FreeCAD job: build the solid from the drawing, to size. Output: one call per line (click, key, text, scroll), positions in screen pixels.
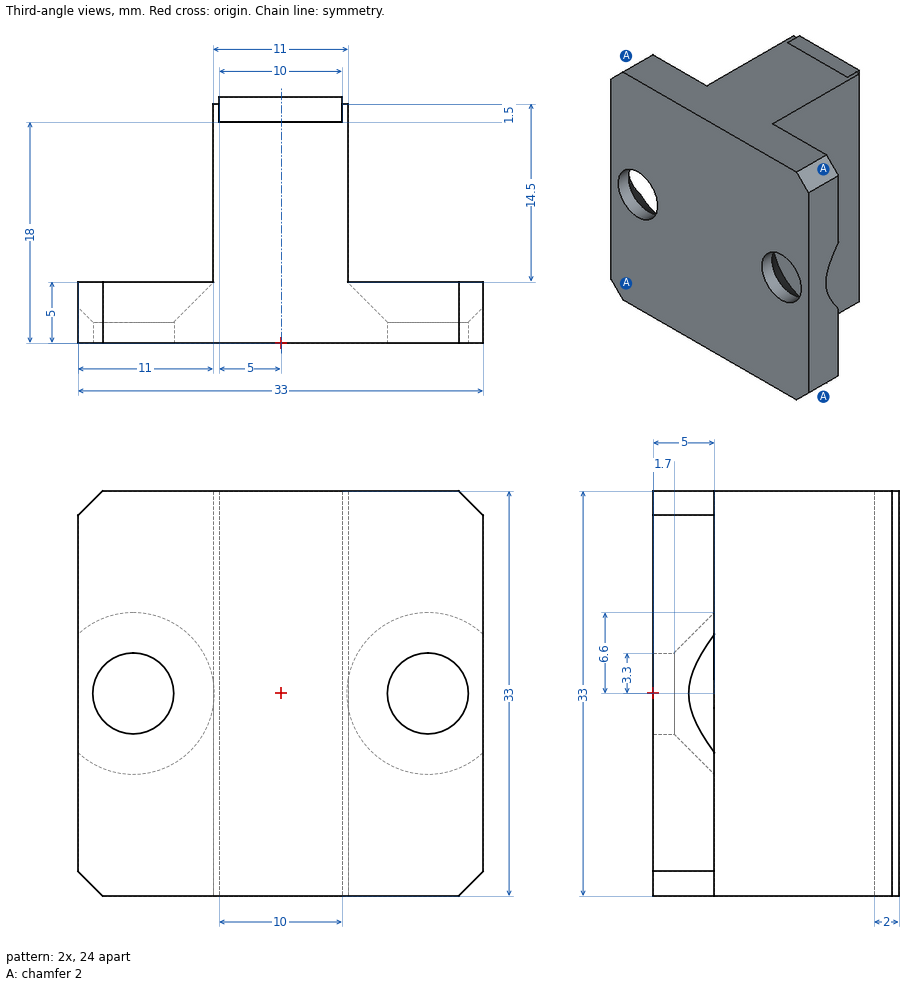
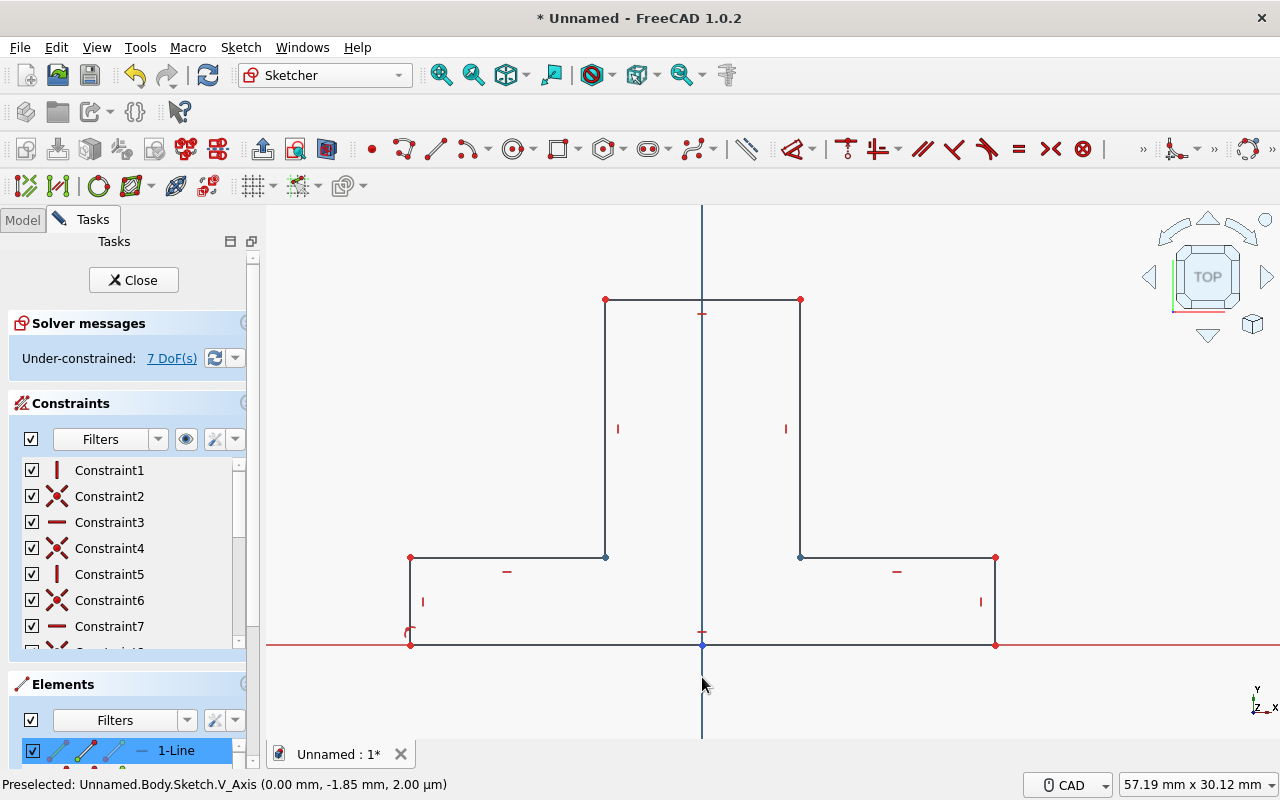
click(1052, 150)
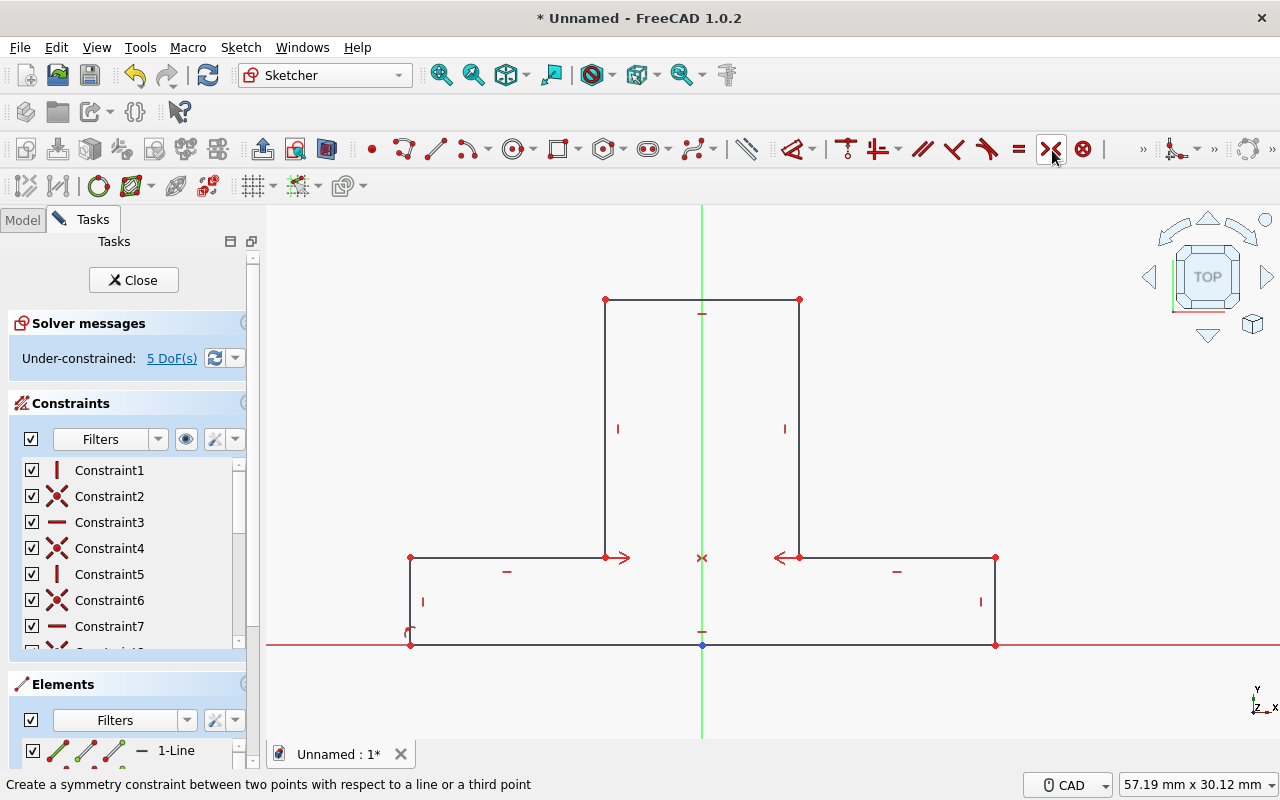
click(792, 150)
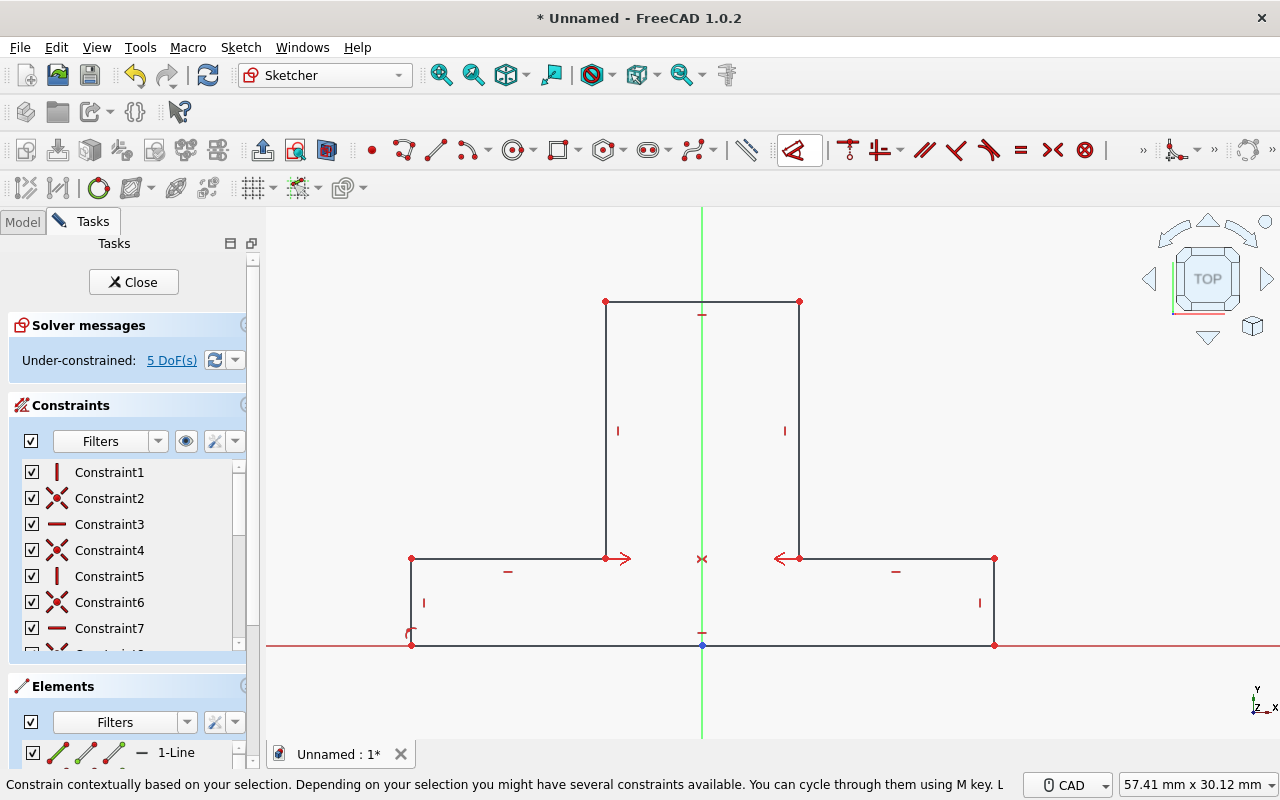
click(411, 585)
click(377, 602)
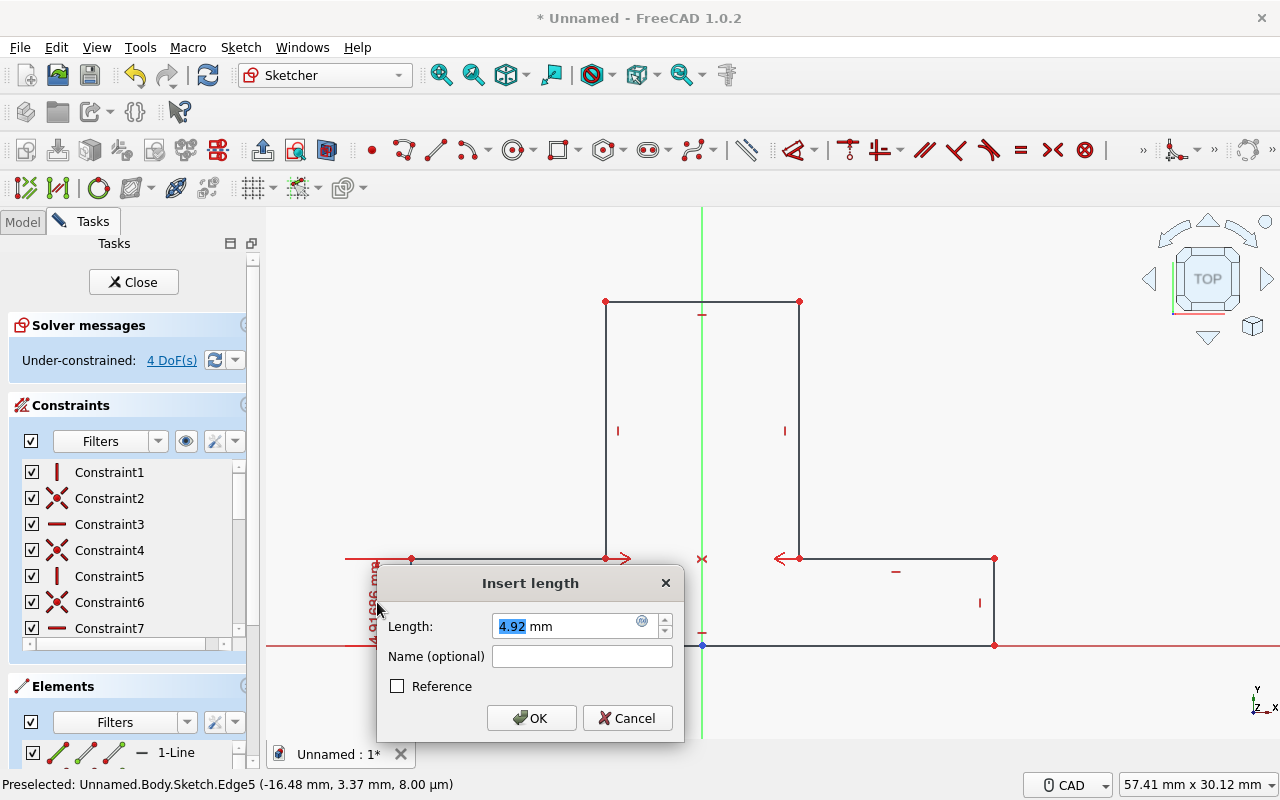
text(5)
key(Return)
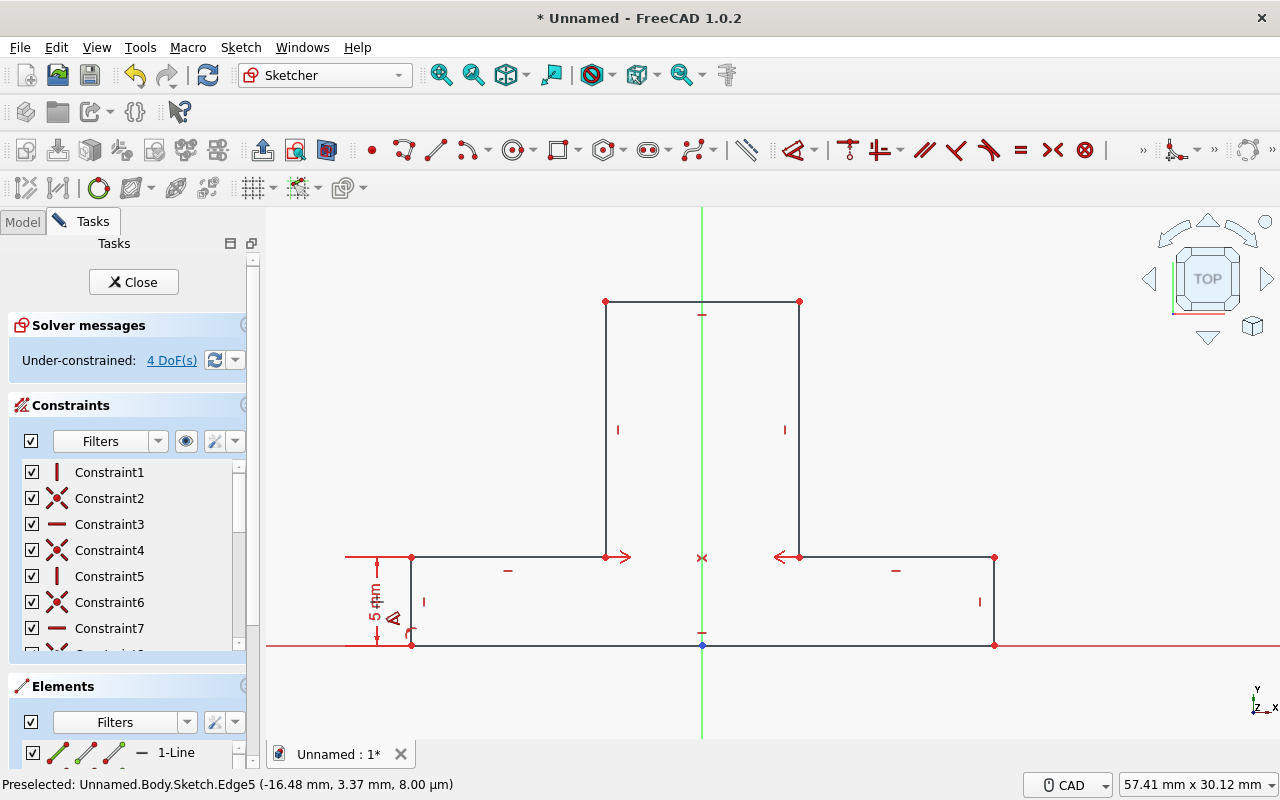
click(741, 302)
click(658, 268)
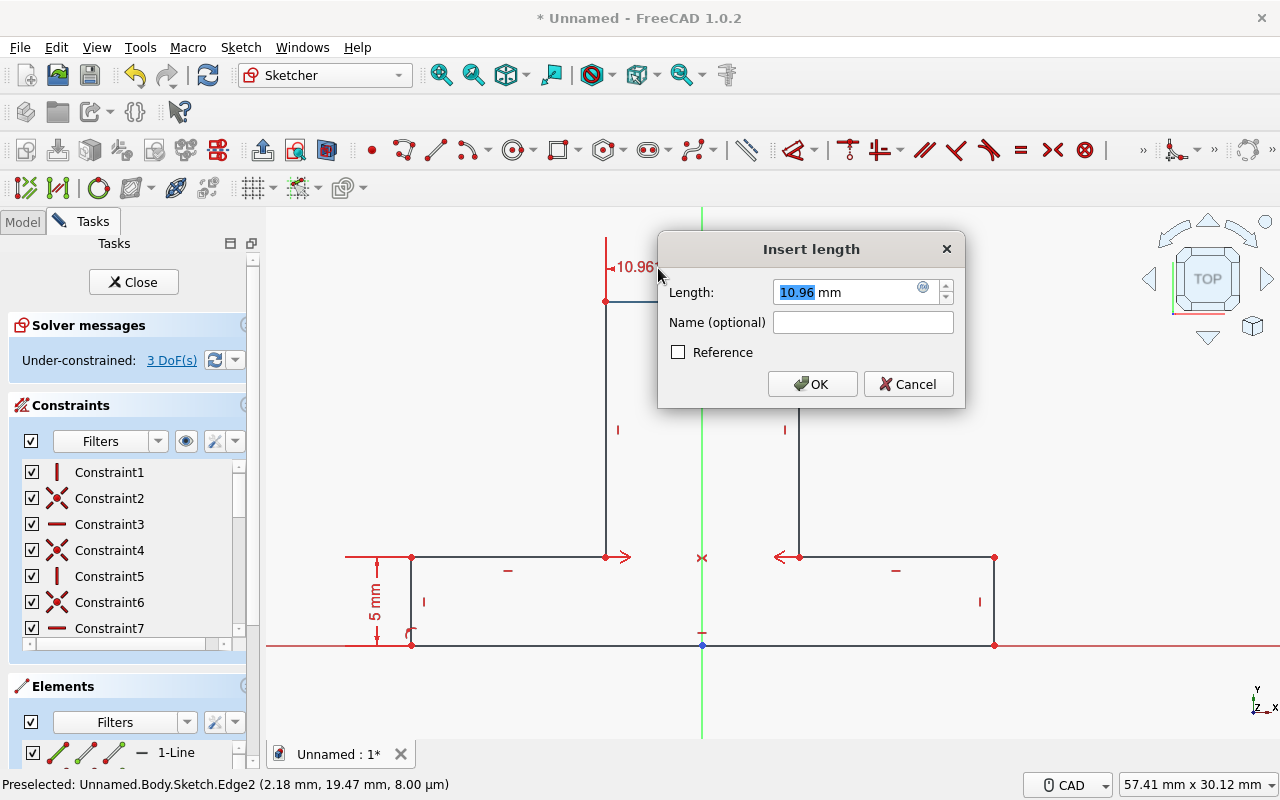
text(11)
key(Return)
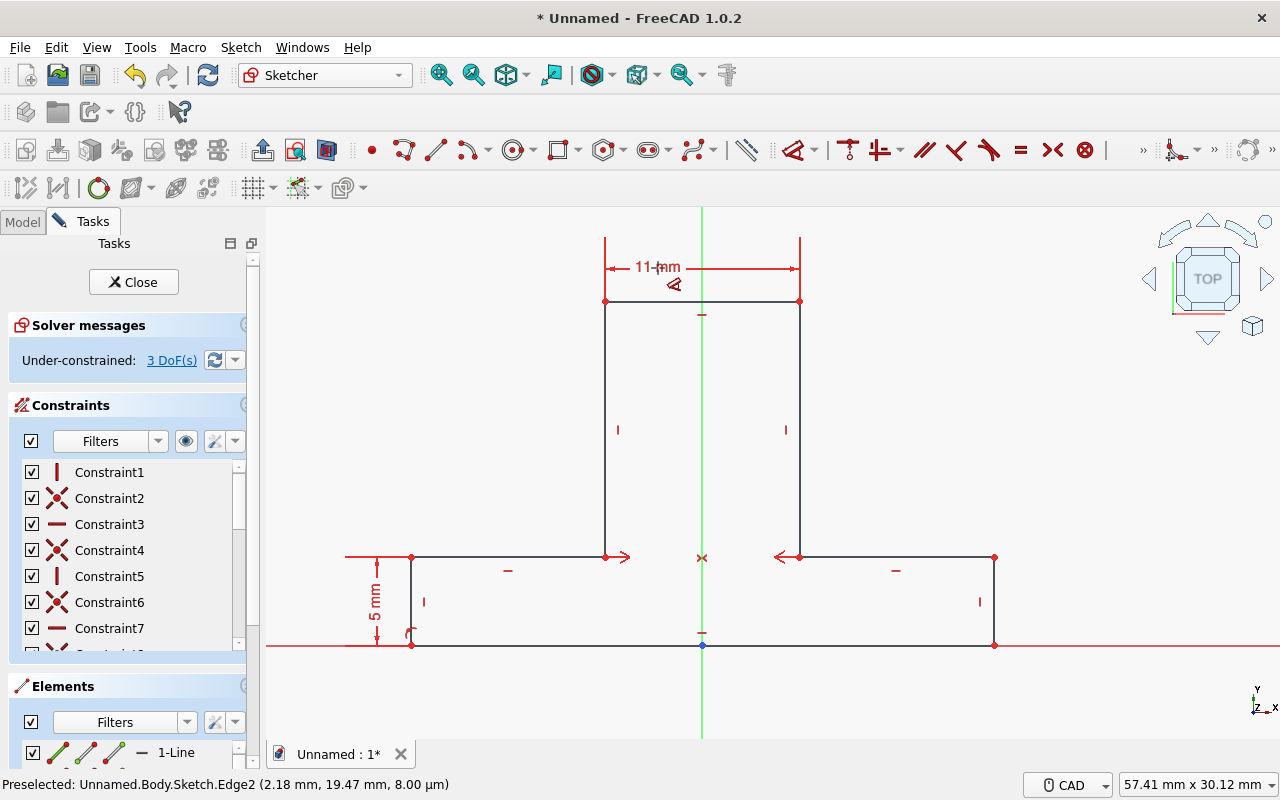
click(547, 557)
click(508, 591)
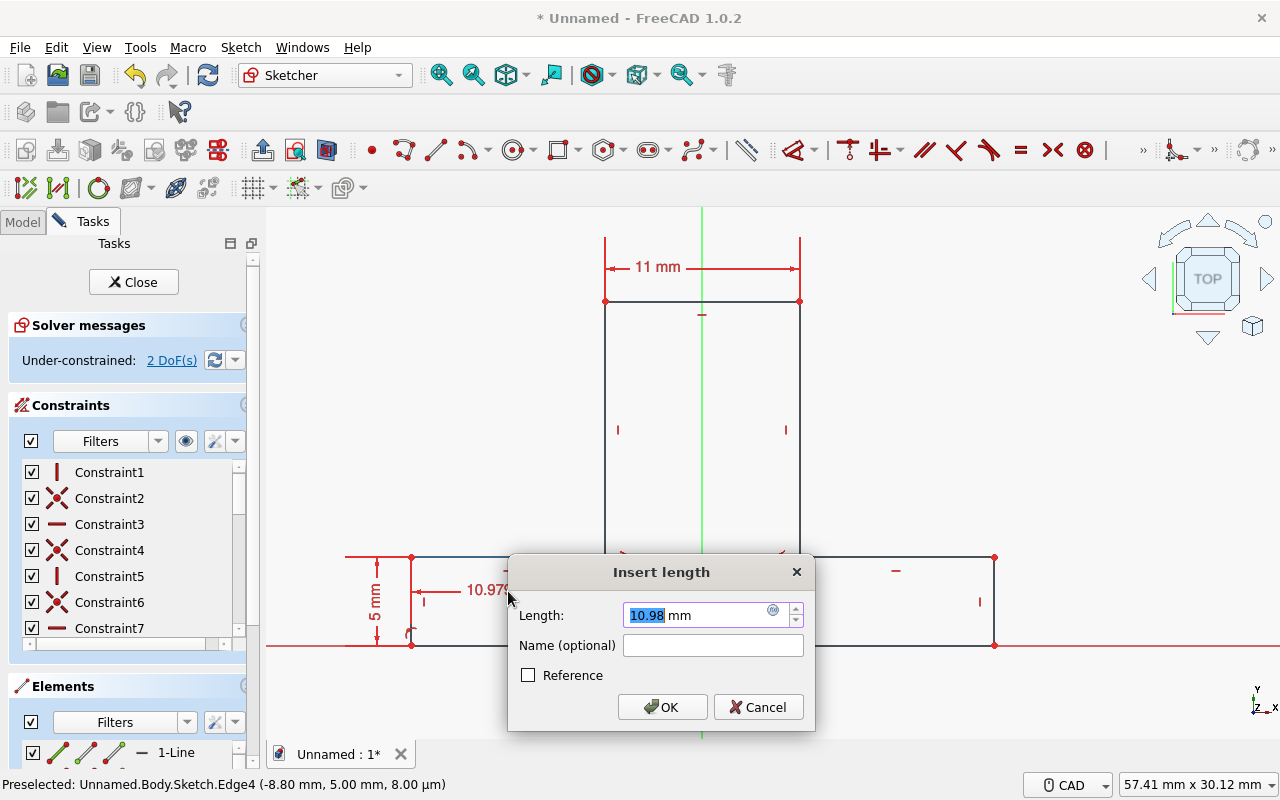
text(11)
key(Return)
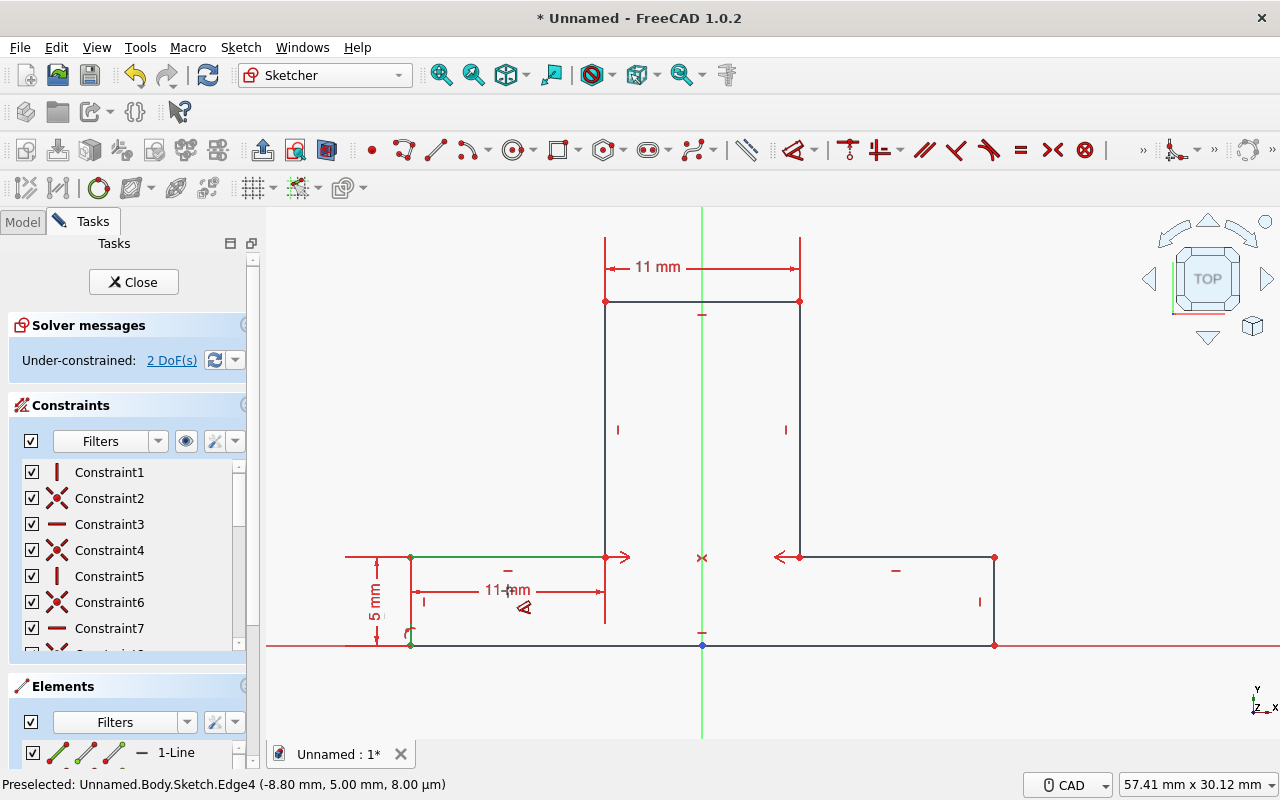
click(586, 646)
click(568, 680)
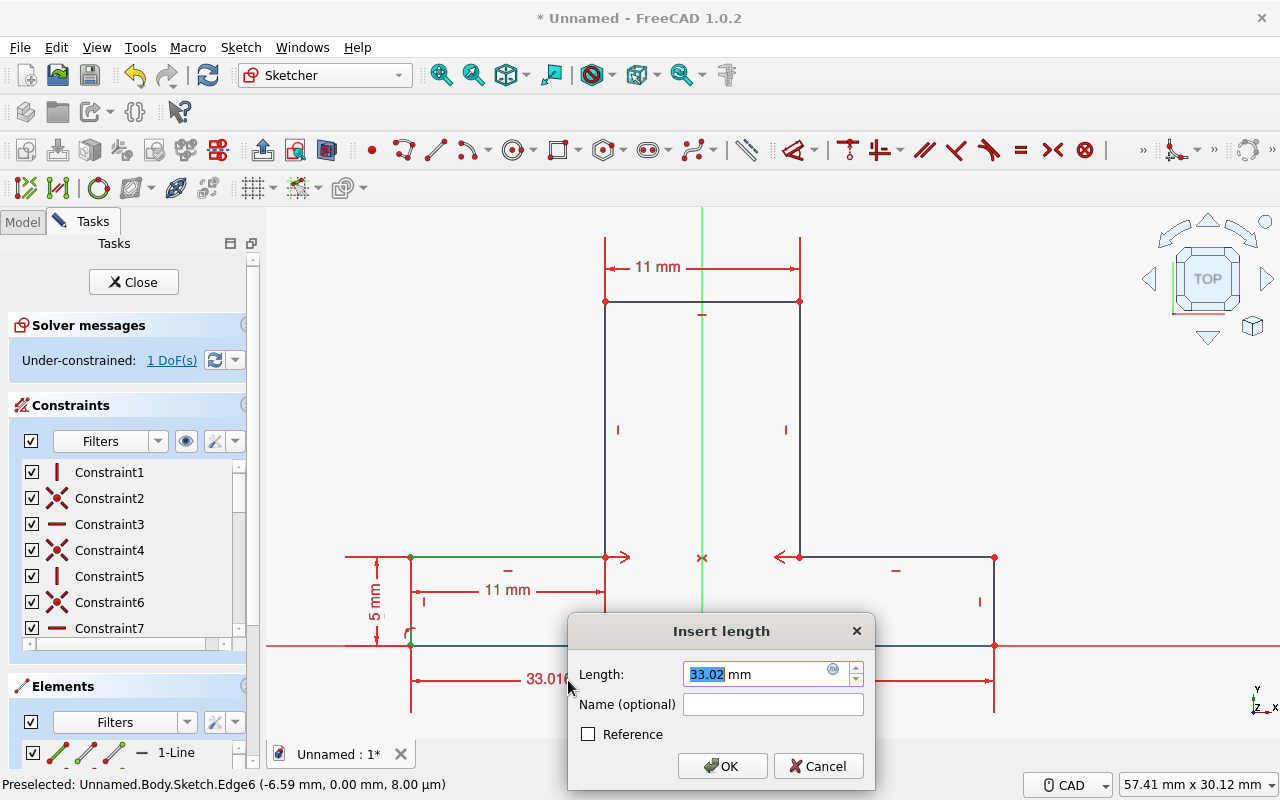
text(33)
key(Return)